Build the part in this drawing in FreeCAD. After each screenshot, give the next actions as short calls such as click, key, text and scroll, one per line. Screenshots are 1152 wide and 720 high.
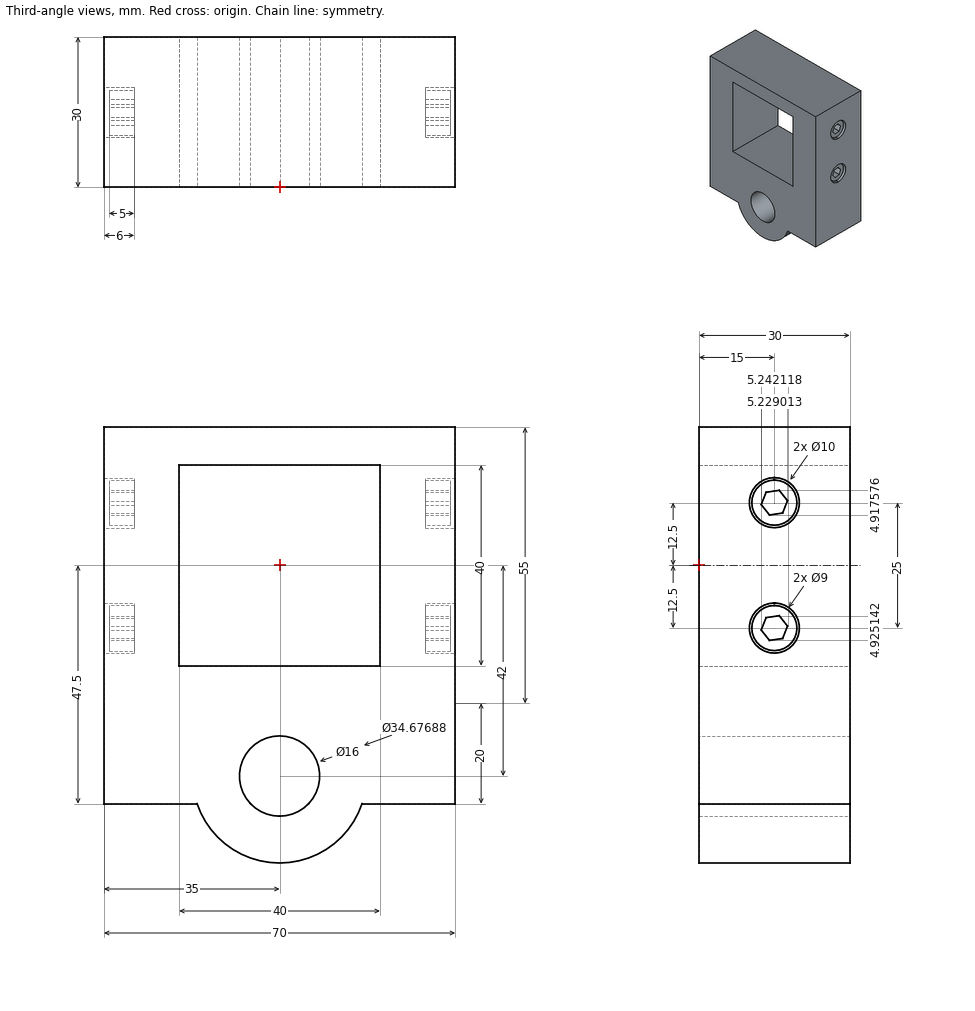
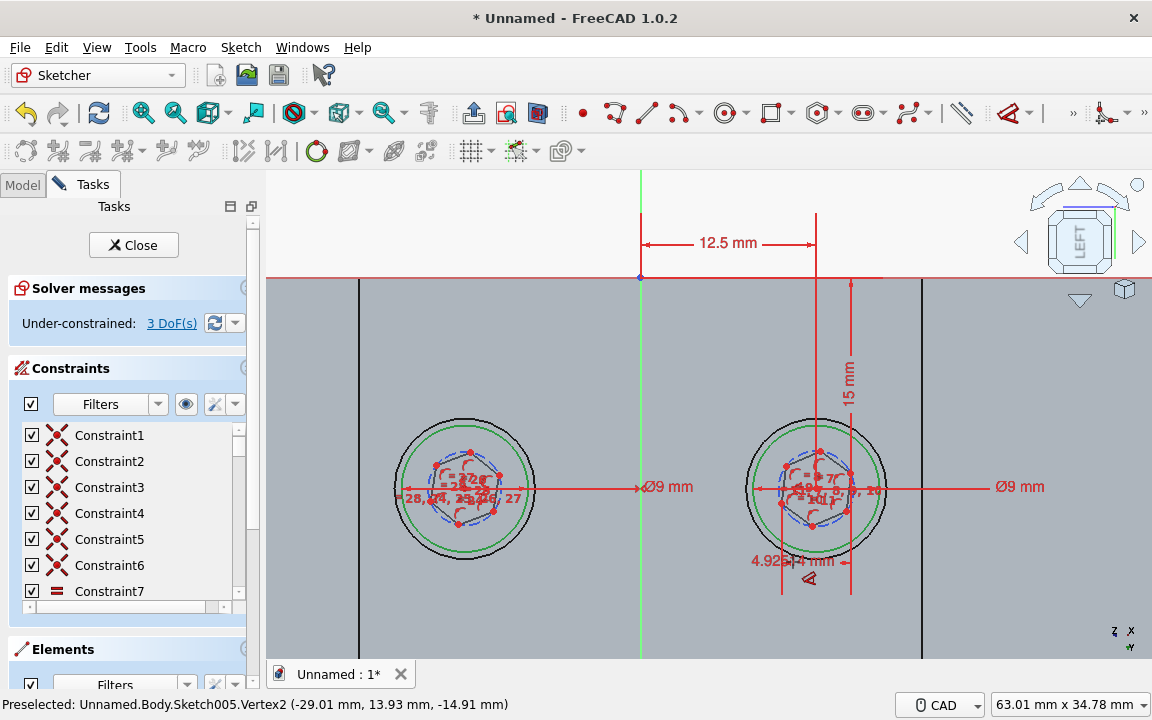
click(812, 526)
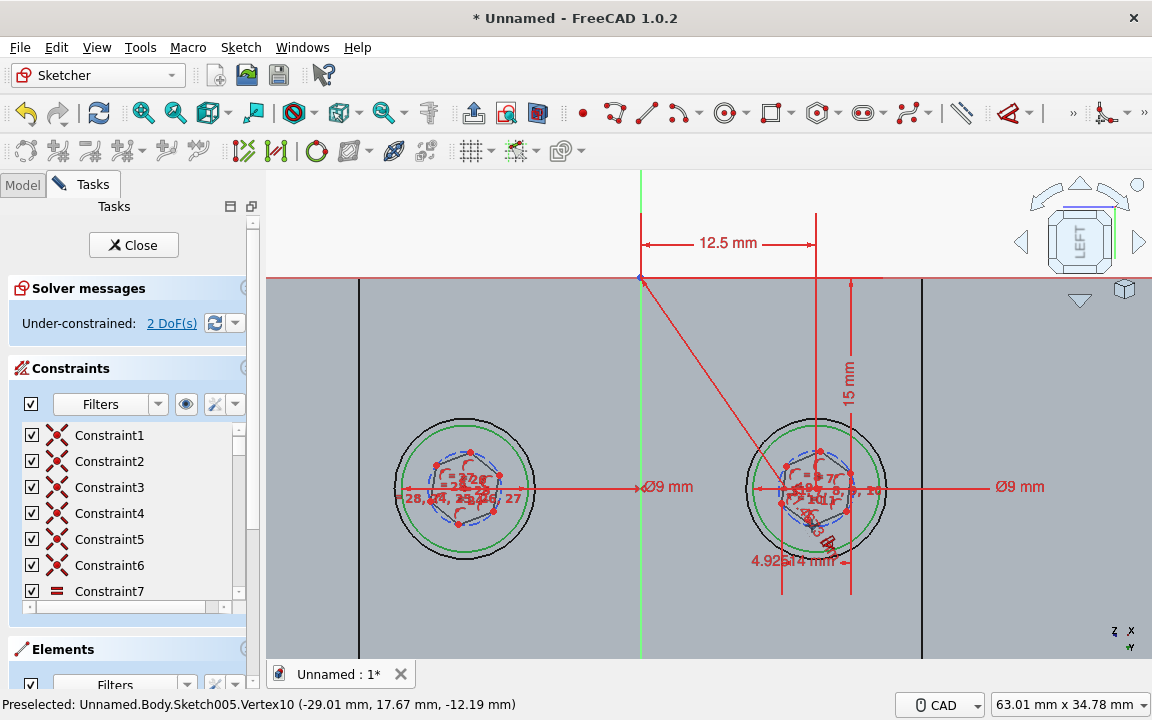
click(821, 451)
click(903, 489)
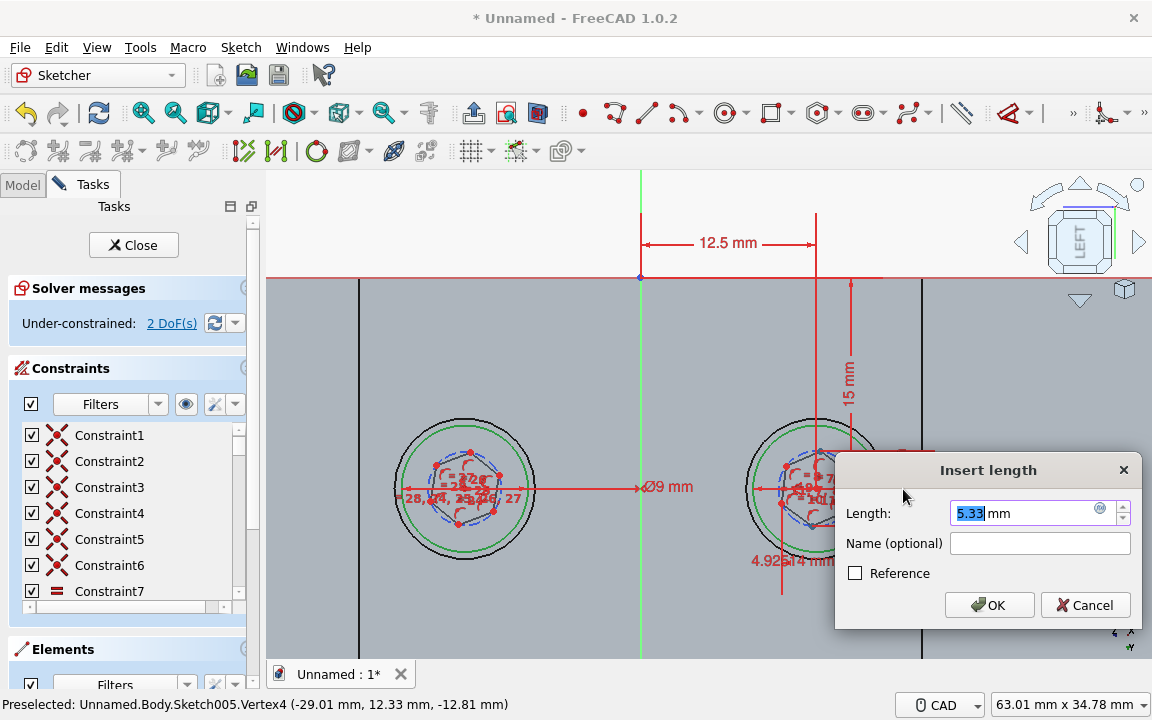
text(5.242118)
key(Return)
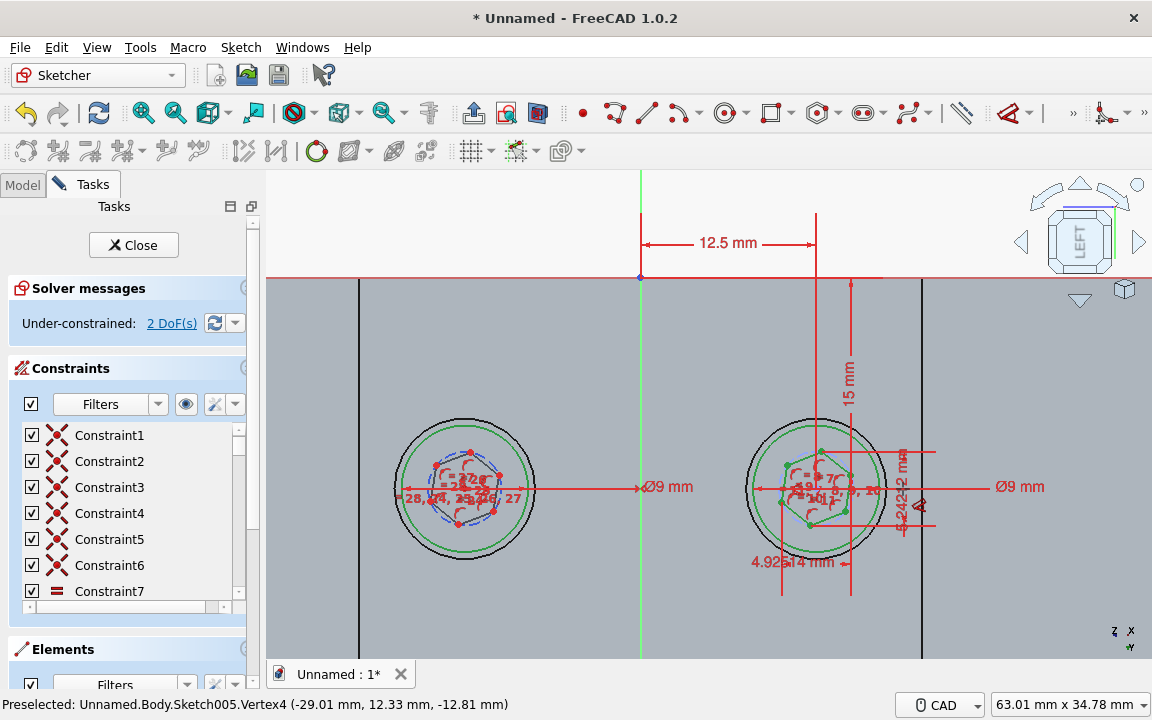
click(431, 502)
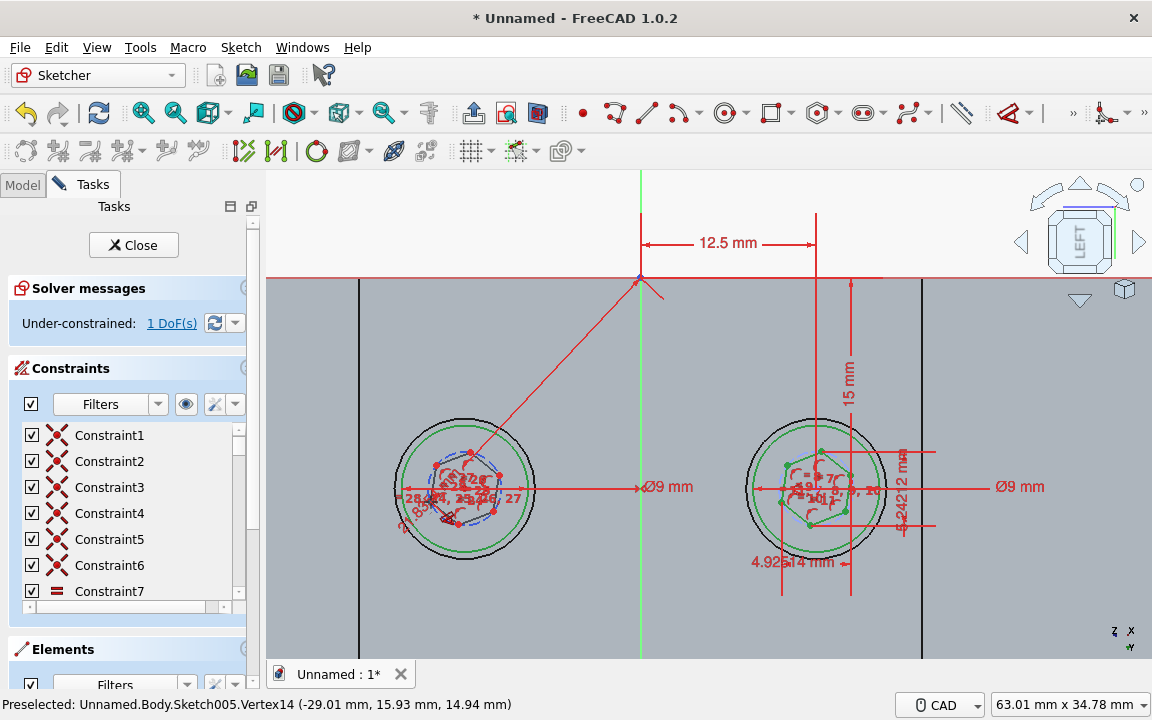
click(499, 476)
click(465, 584)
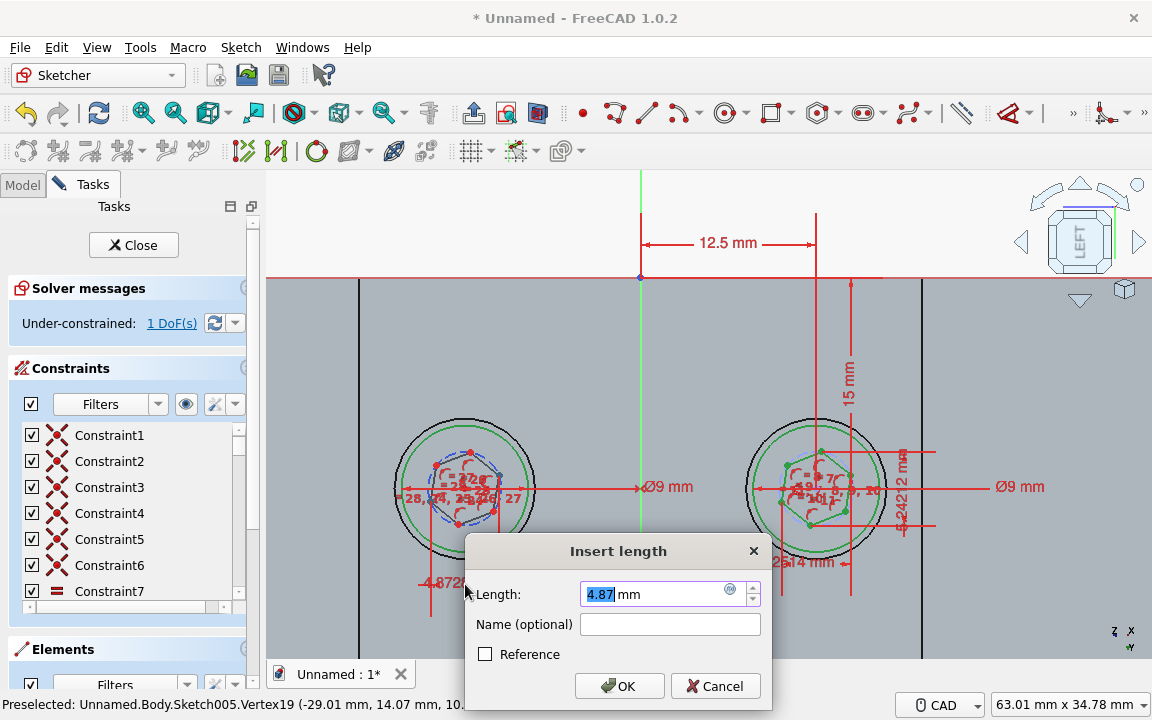
text(4.917576)
key(Return)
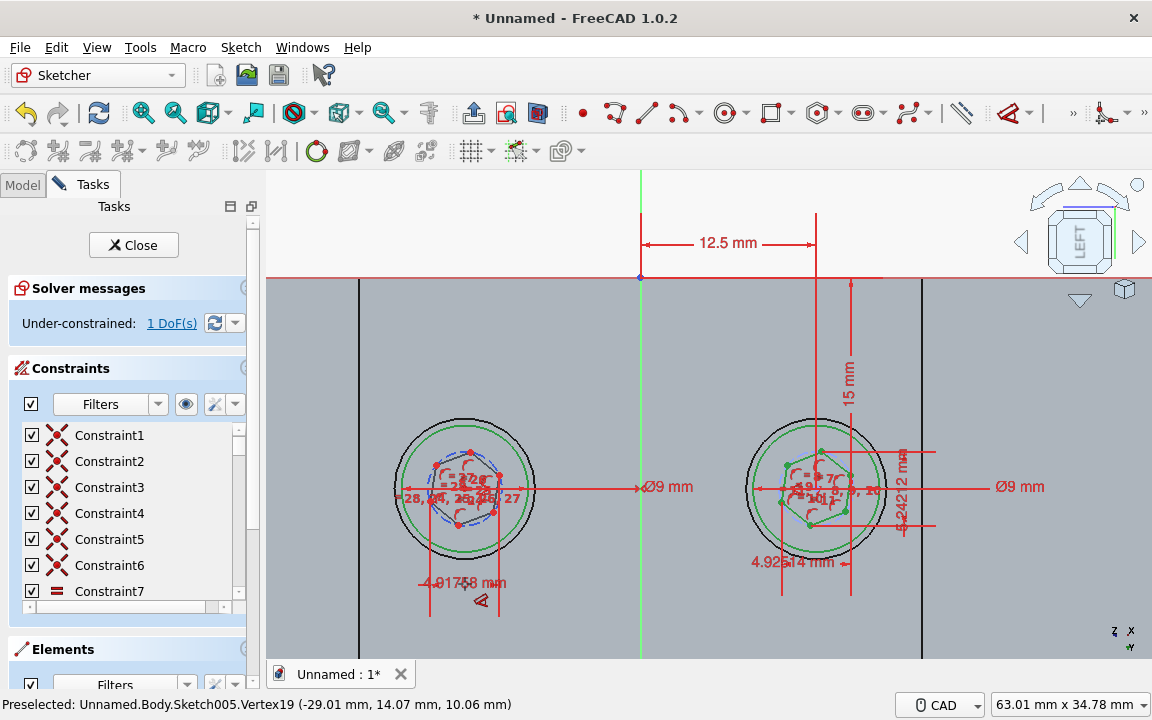
click(459, 525)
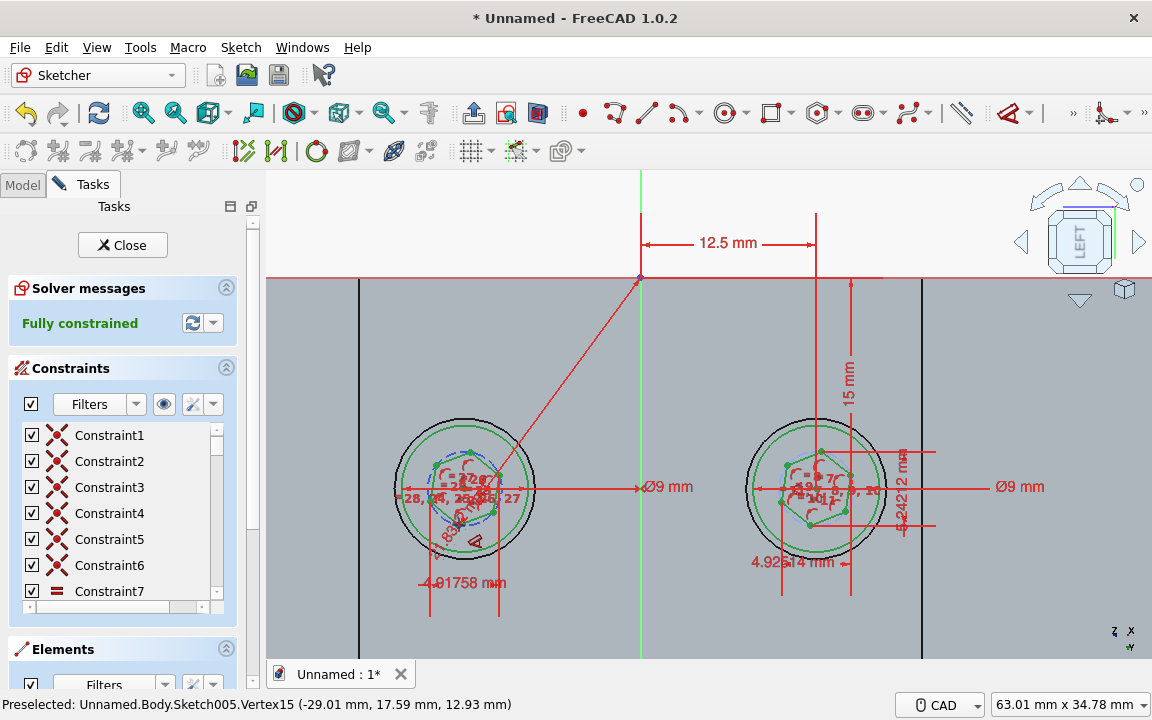
click(471, 452)
click(377, 489)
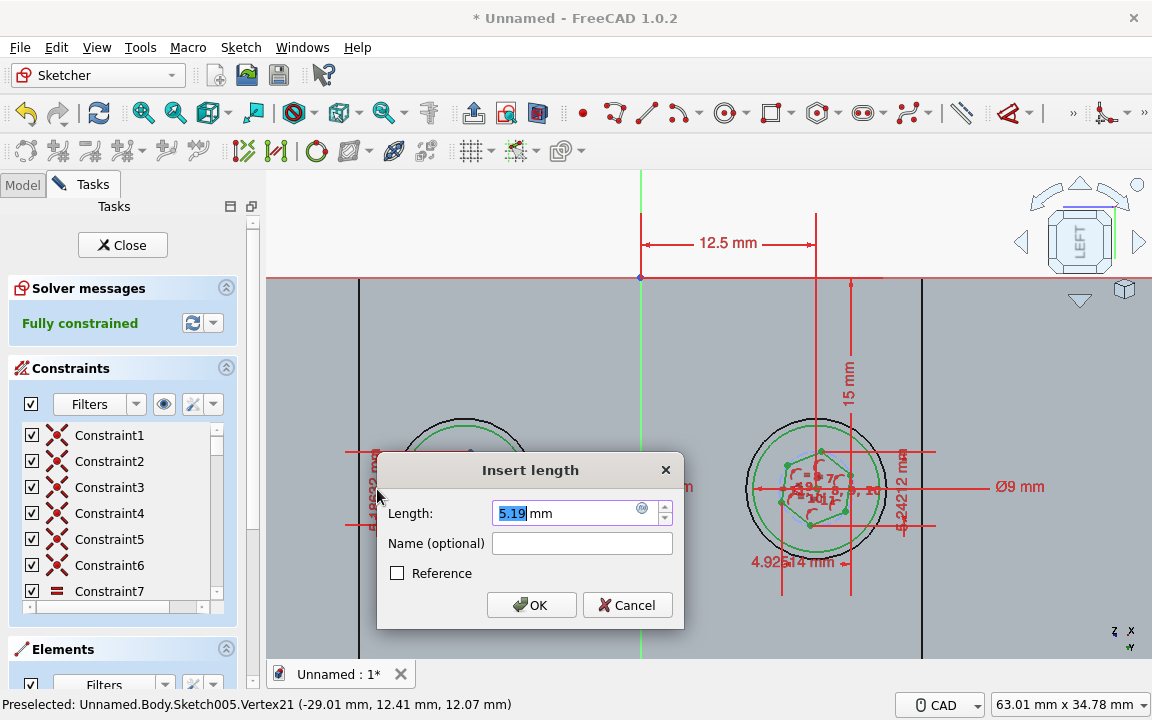
text(5.229013)
key(Return)
key(Escape)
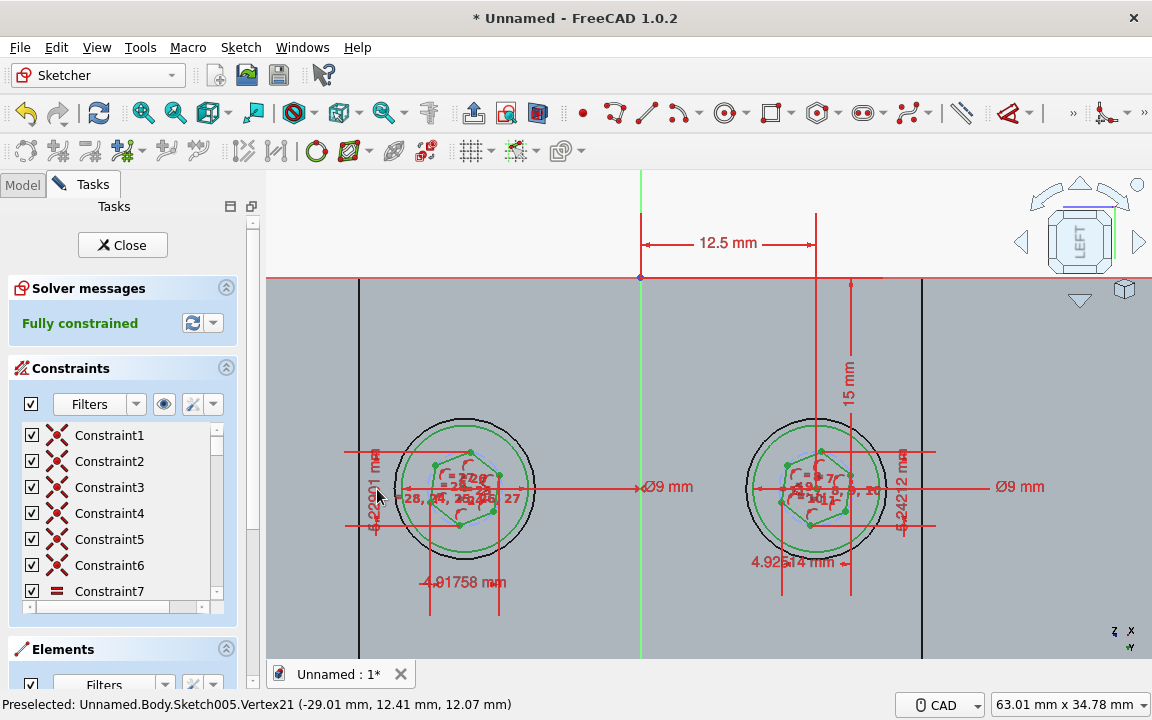
click(123, 245)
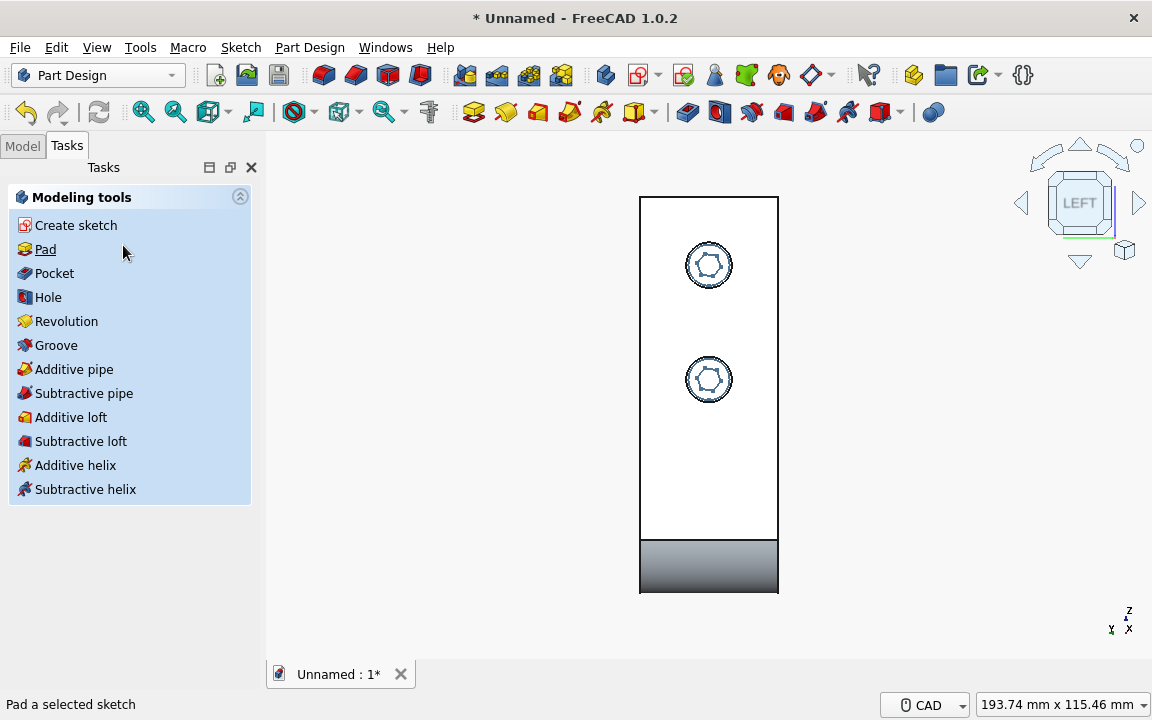
click(474, 112)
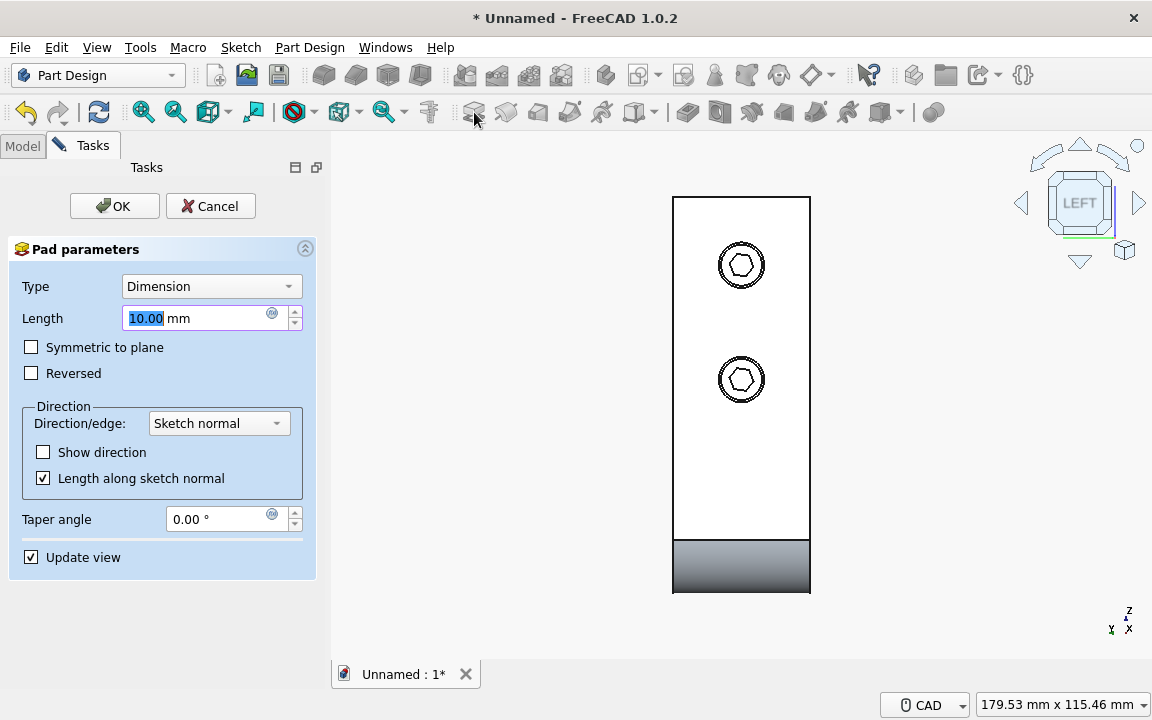
text(5)
key(Tab)